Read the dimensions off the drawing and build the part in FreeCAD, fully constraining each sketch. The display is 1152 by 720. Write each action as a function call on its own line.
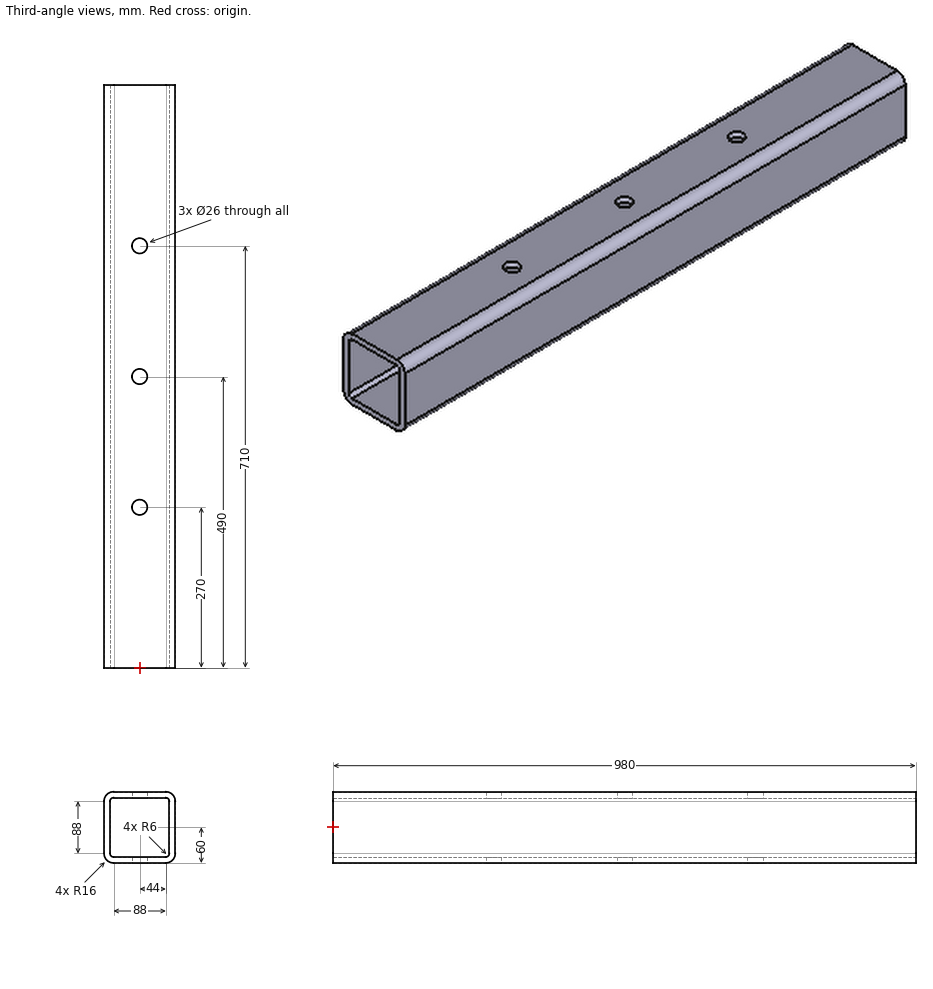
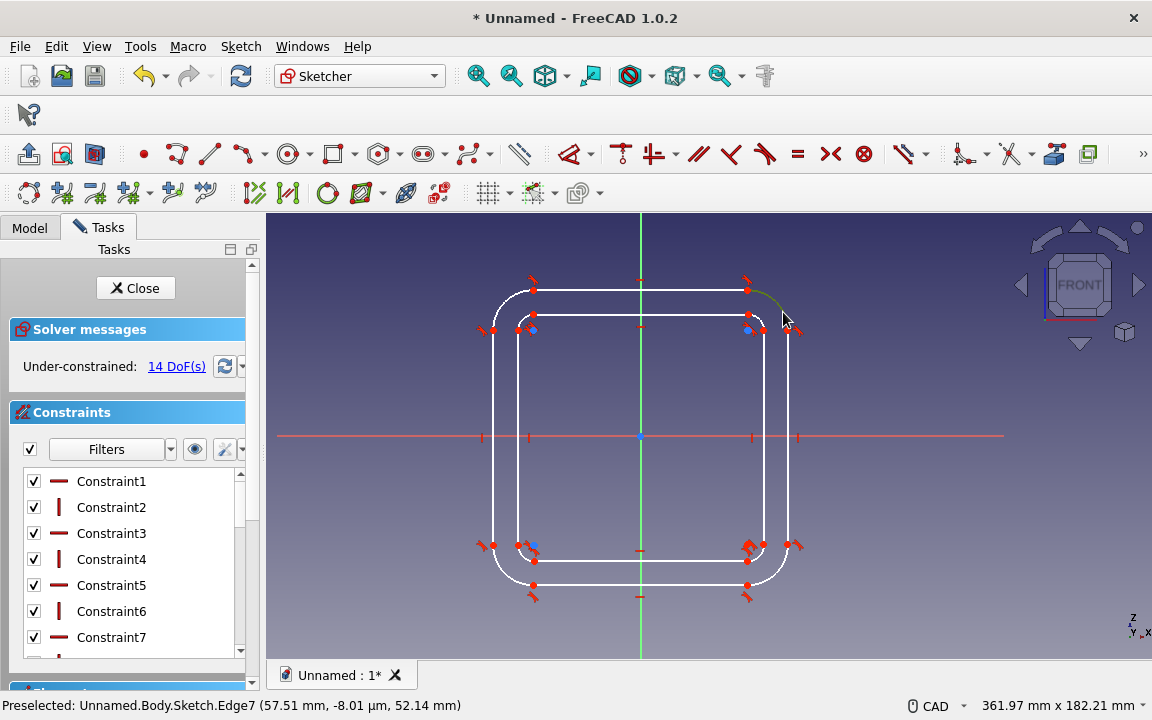
click(759, 319)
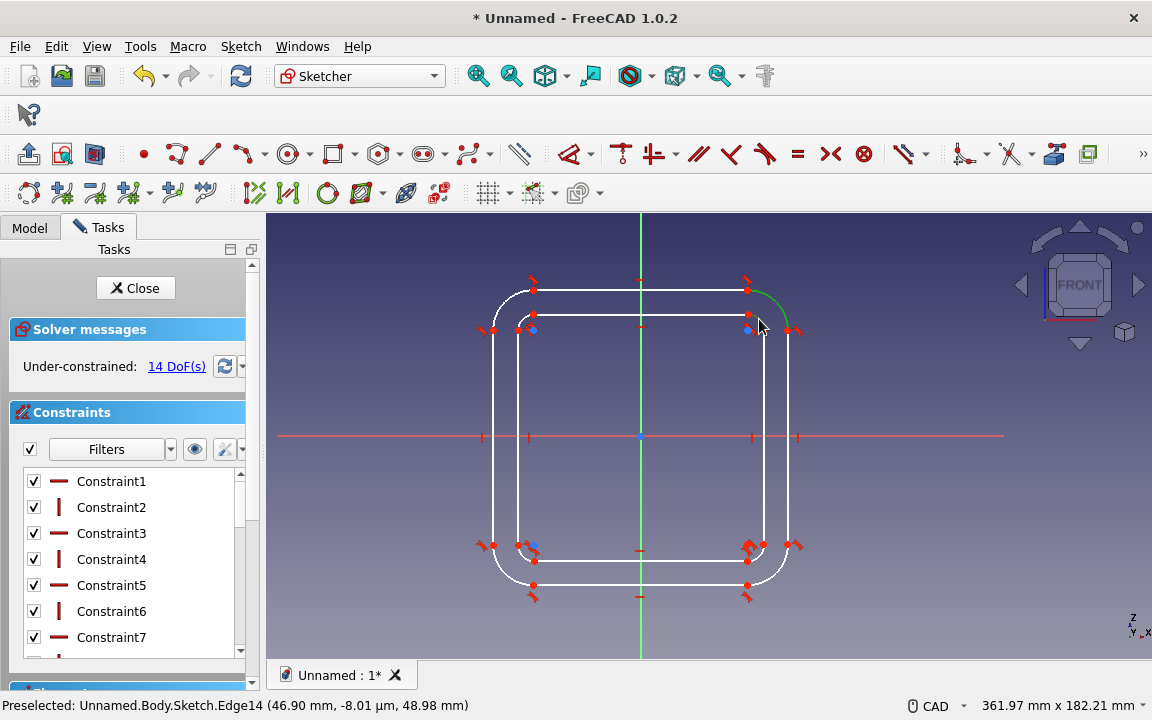
click(621, 154)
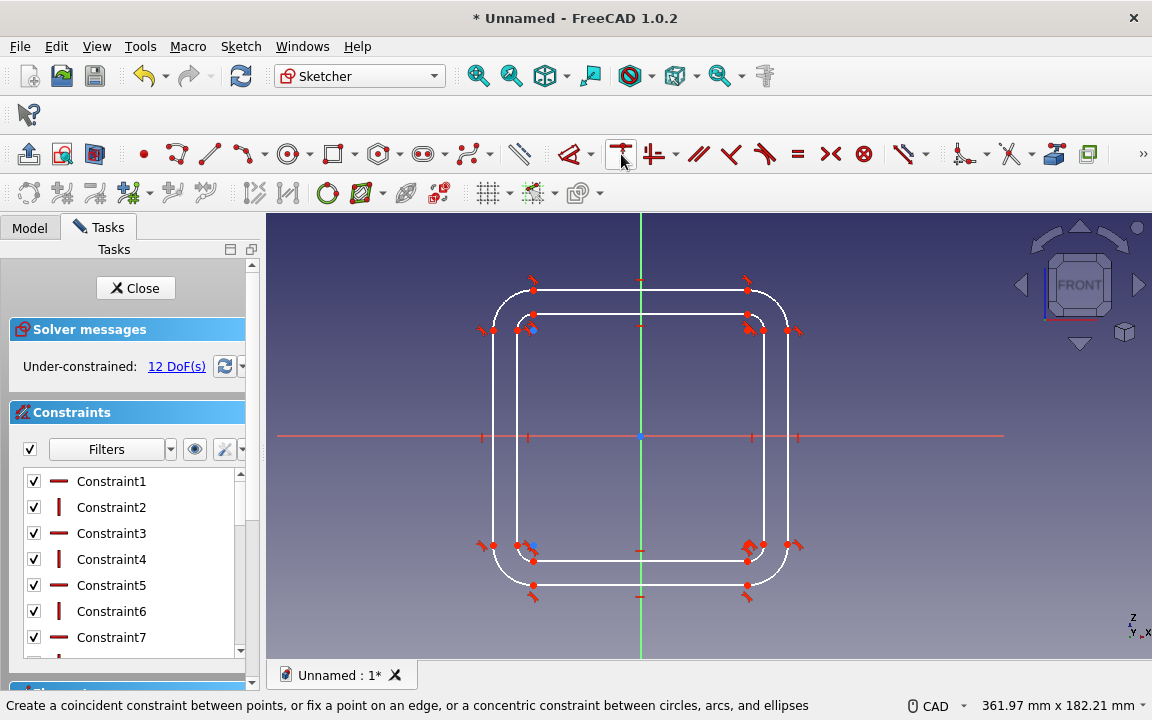
click(515, 295)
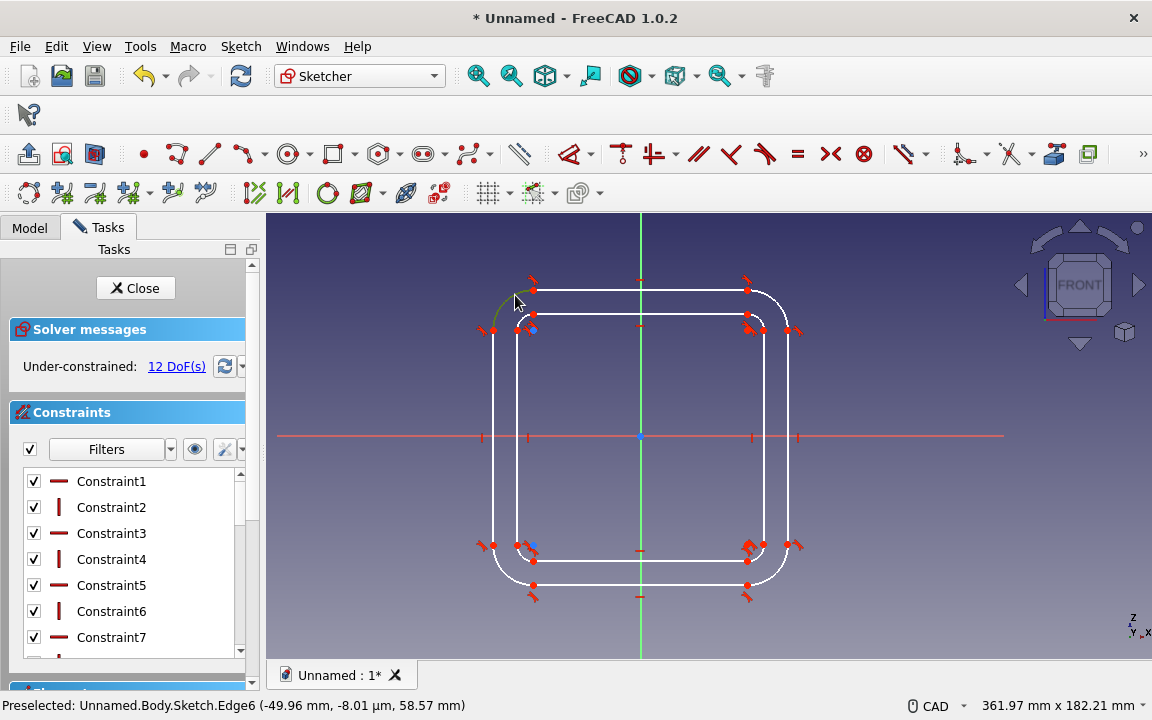
click(522, 319)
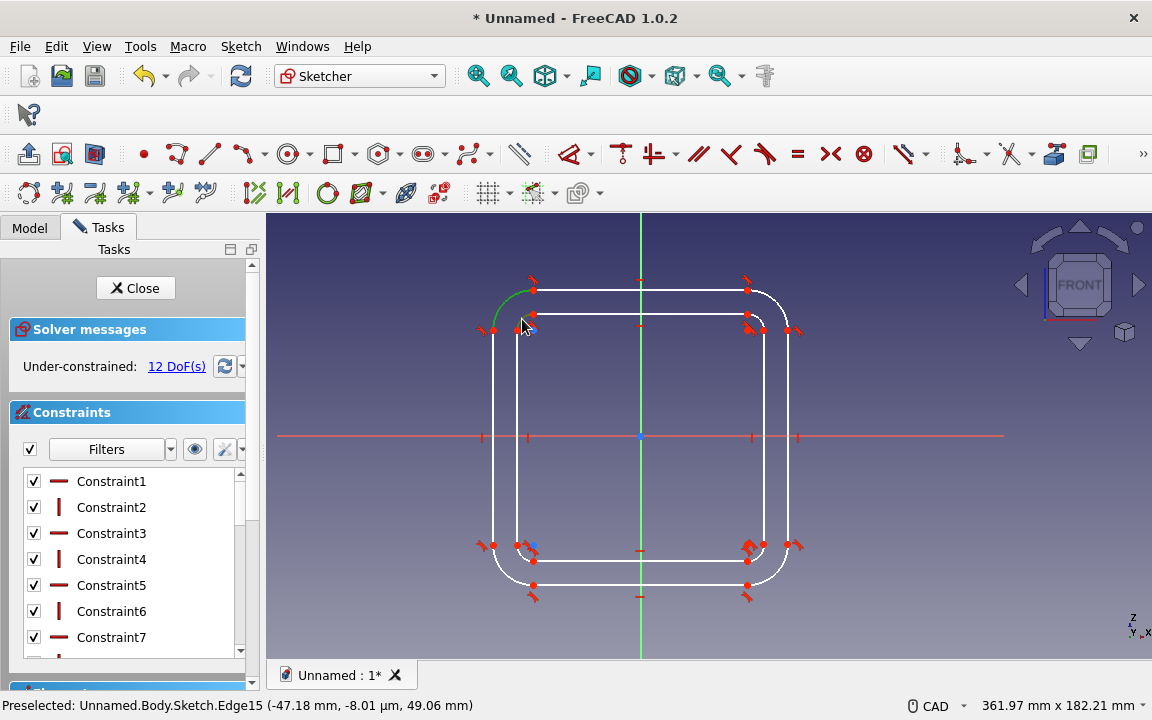
click(621, 154)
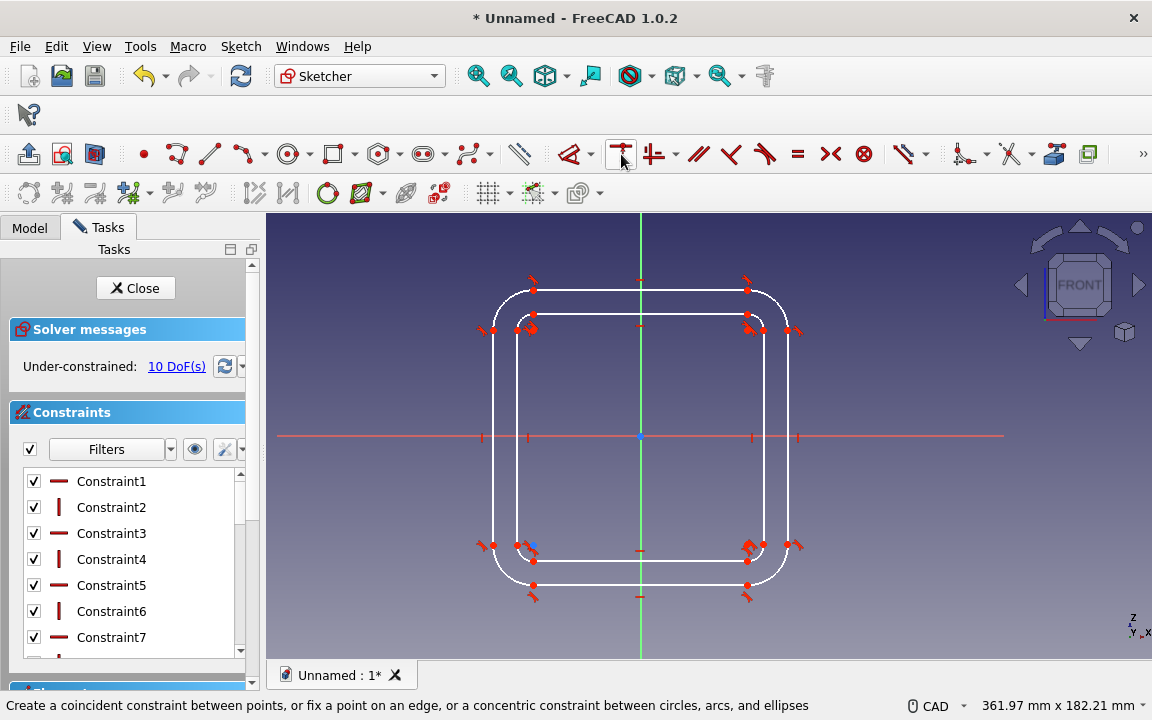
click(498, 563)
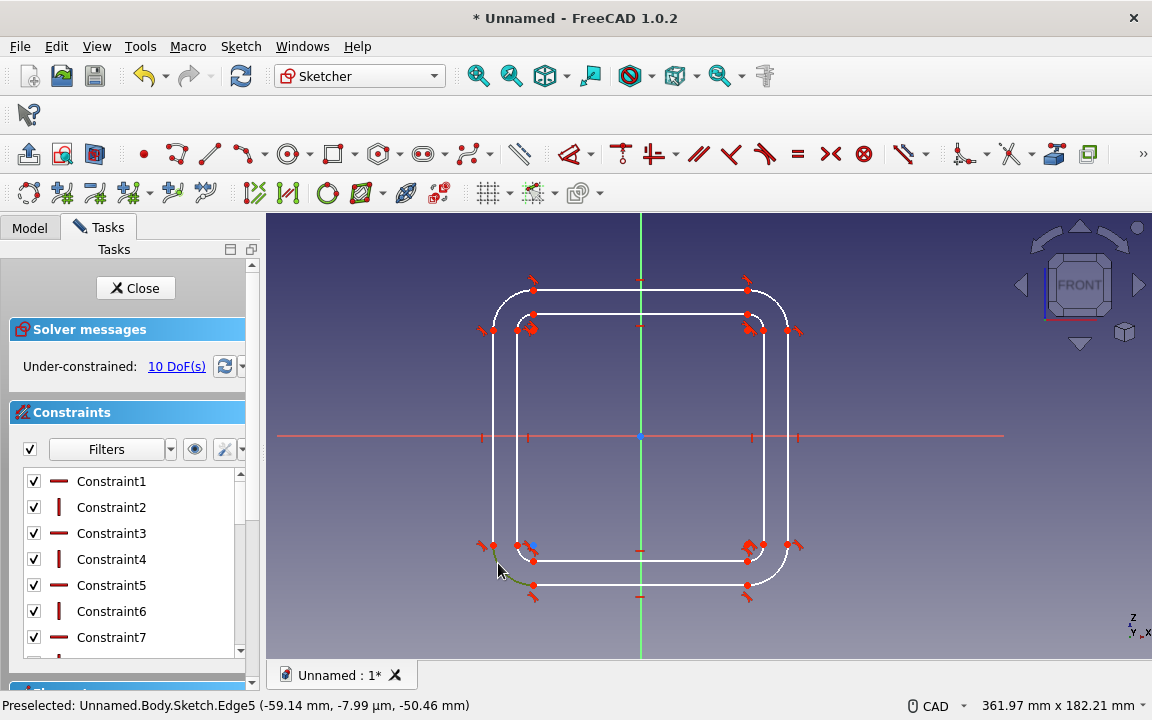
click(515, 295)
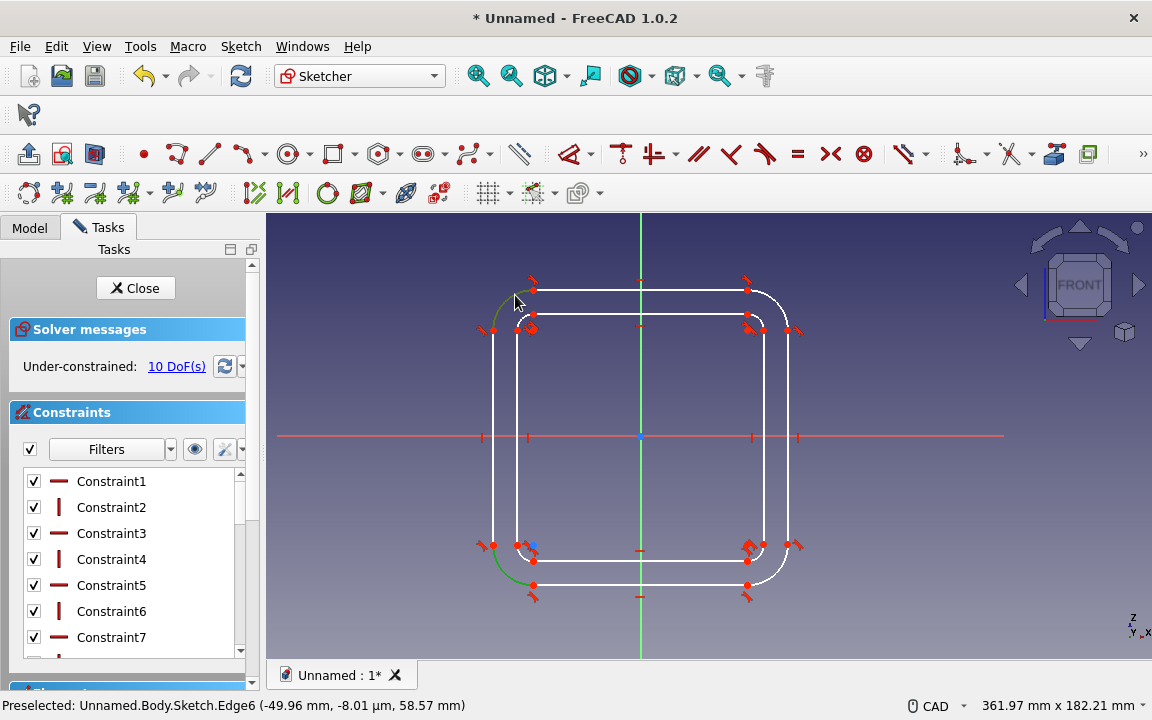
click(783, 312)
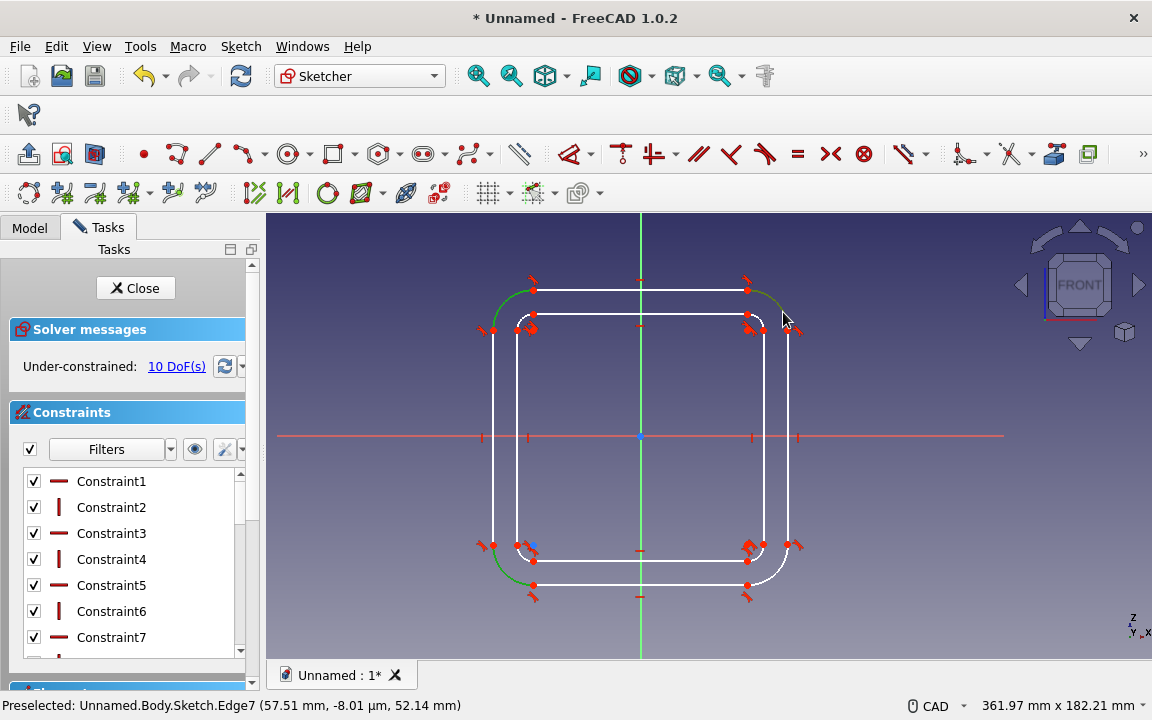
click(766, 581)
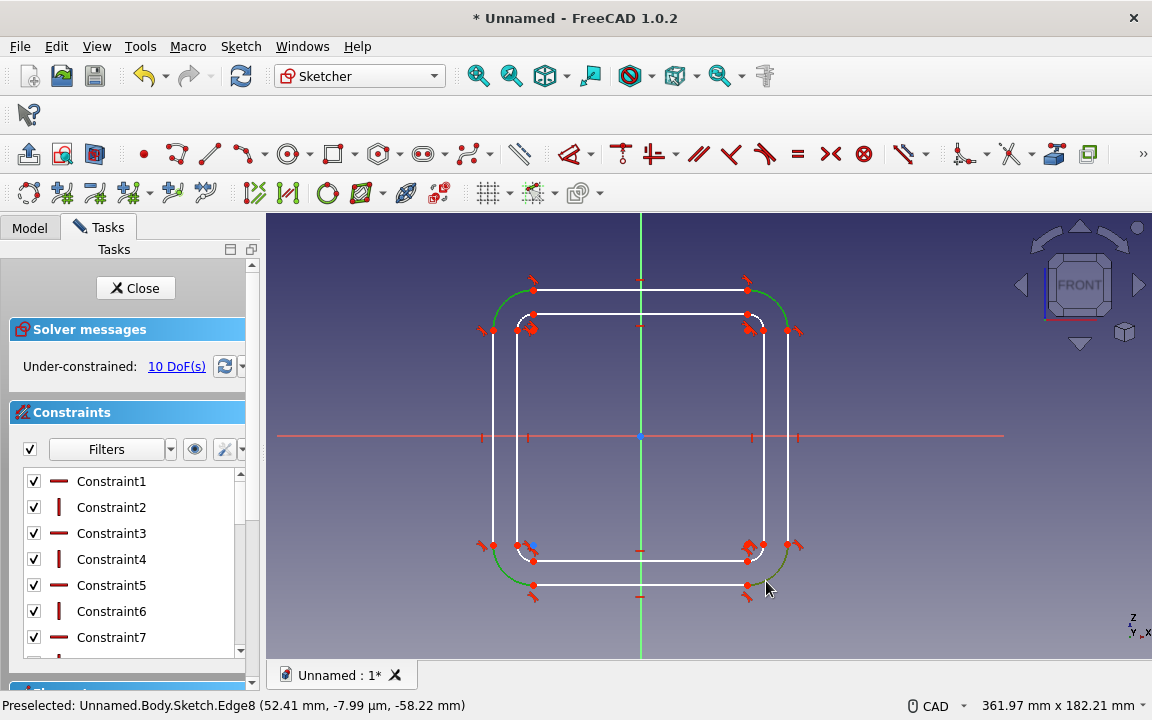
click(798, 154)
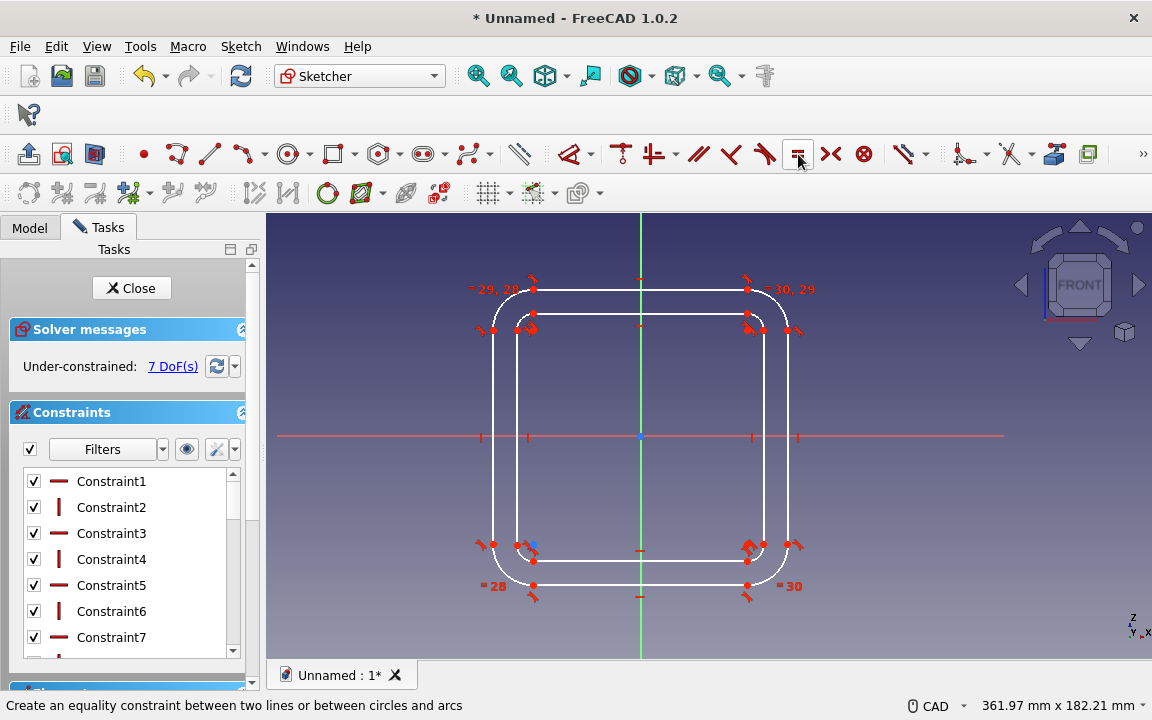
click(759, 556)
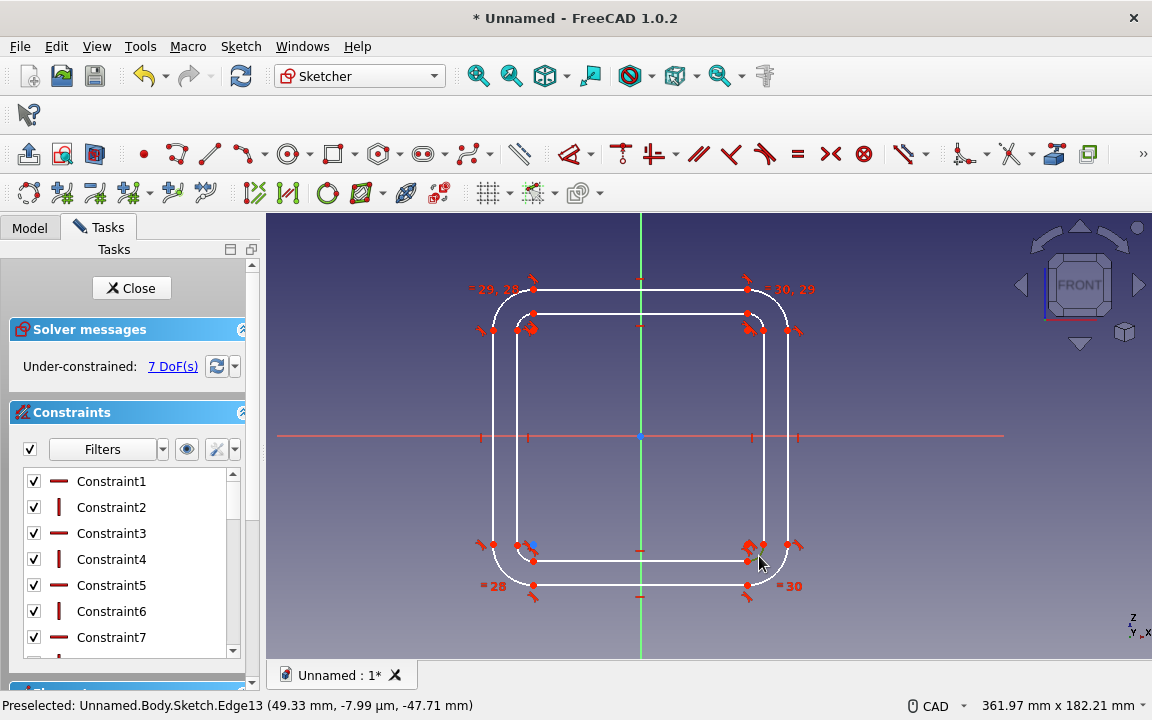
click(522, 557)